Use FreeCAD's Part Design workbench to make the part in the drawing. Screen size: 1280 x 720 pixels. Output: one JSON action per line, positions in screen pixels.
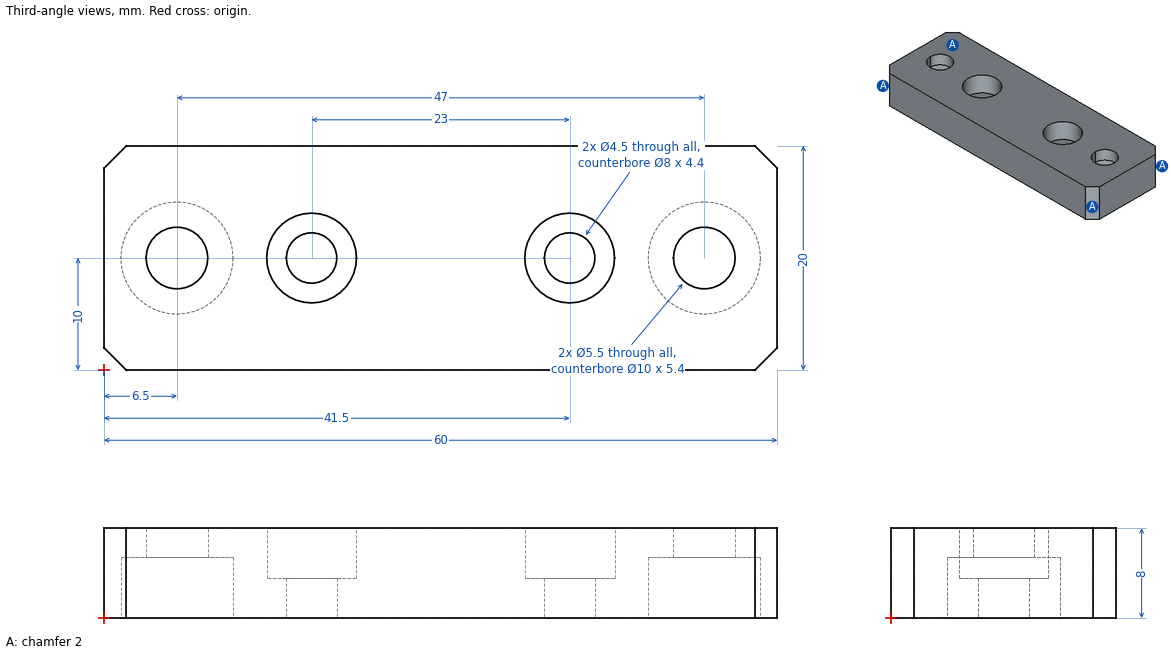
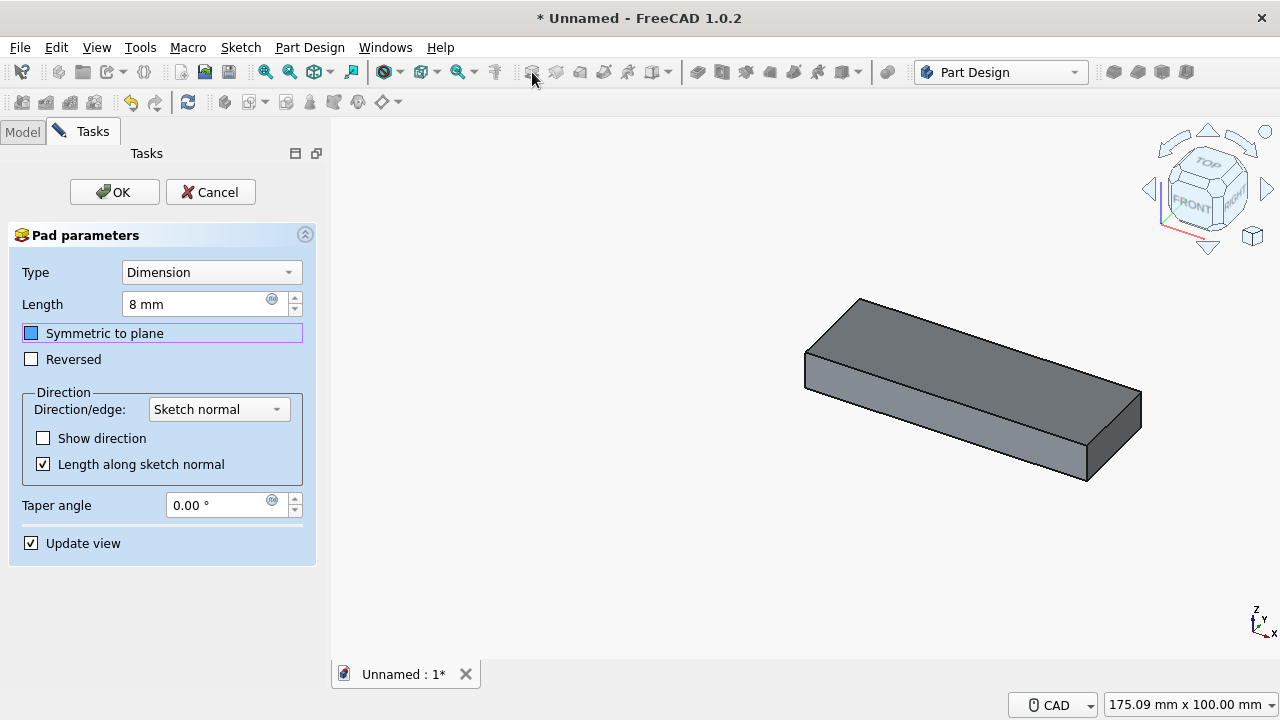
{"action": "left_click", "coordinate": [115, 192]}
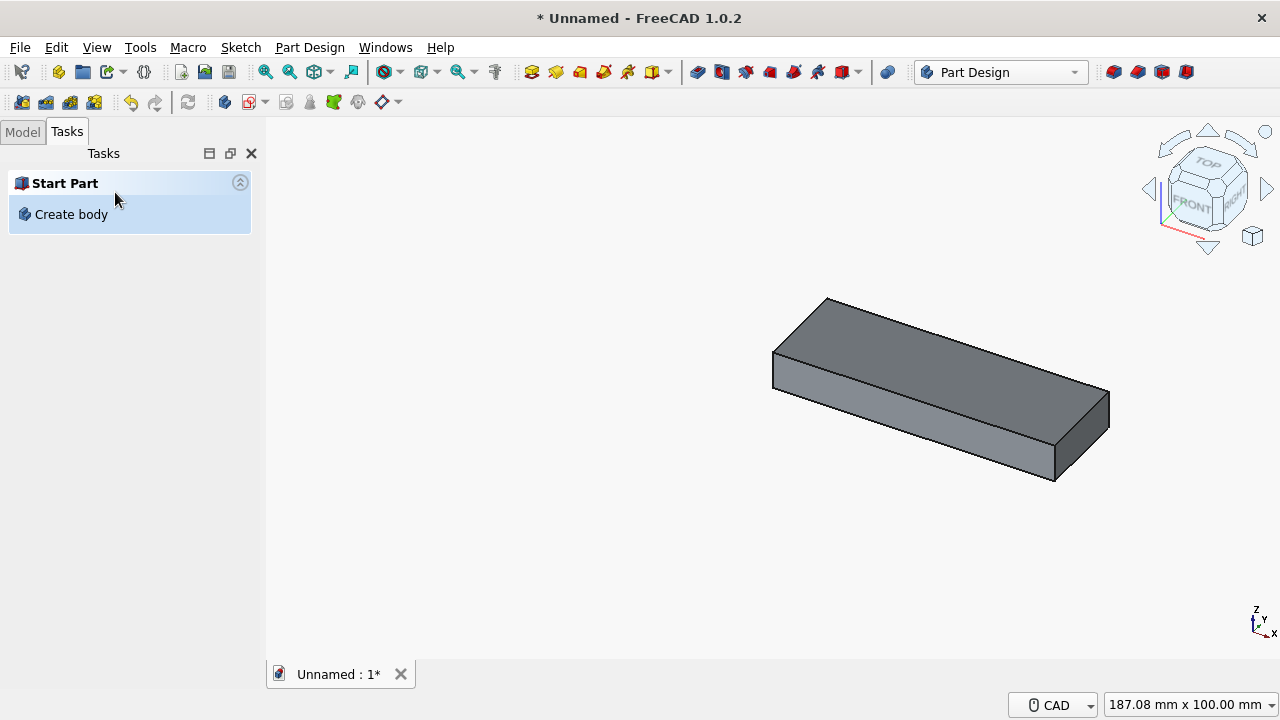
{"action": "key", "text": "v f"}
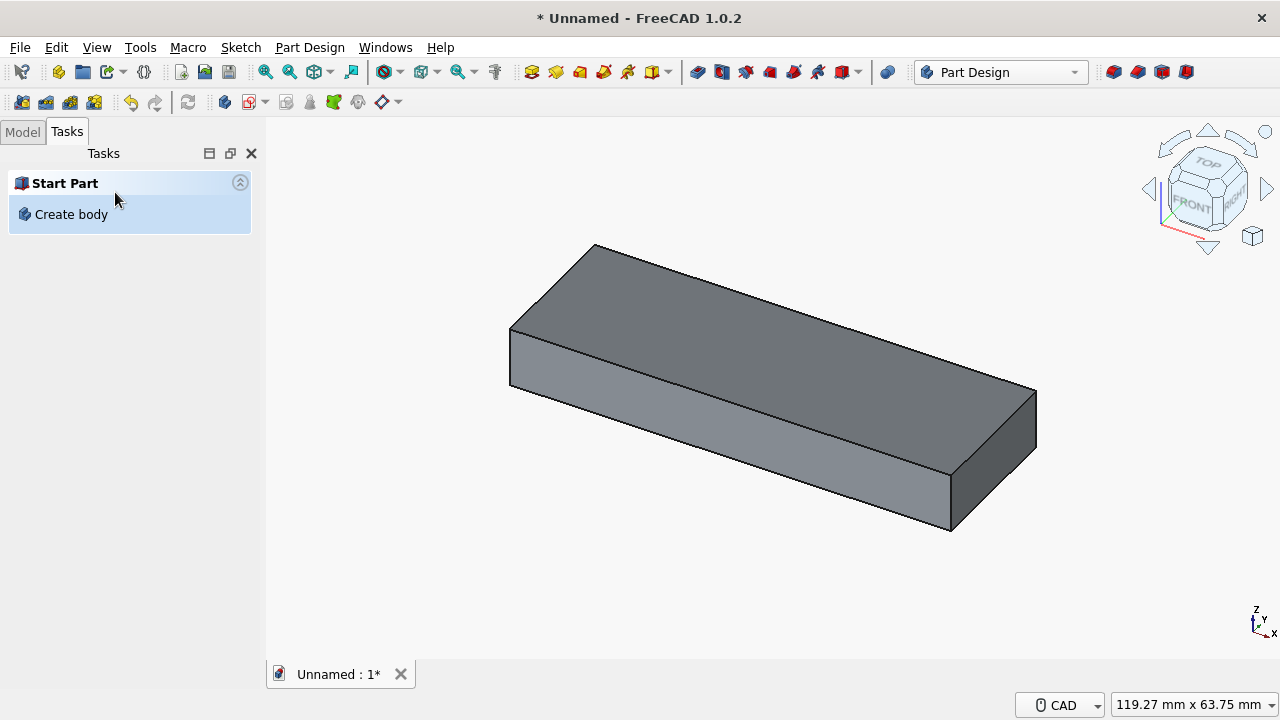
{"action": "left_click", "coordinate": [899, 401]}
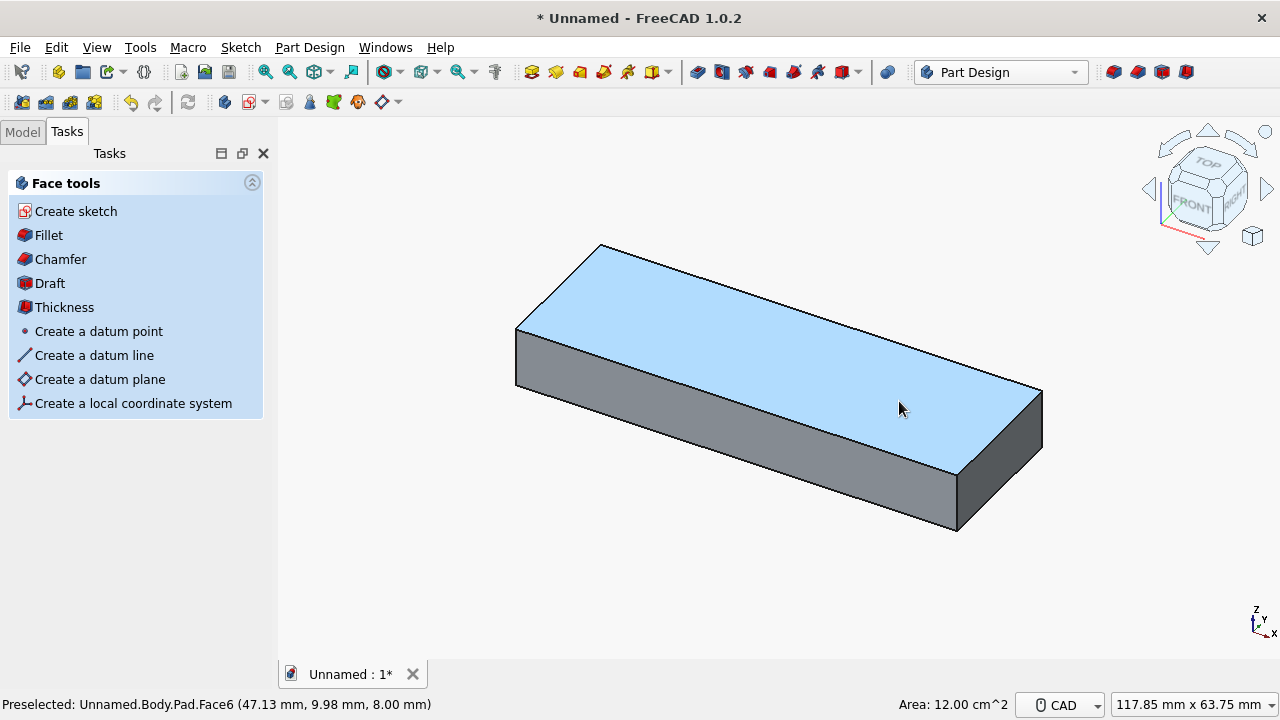
{"action": "left_click", "coordinate": [250, 102]}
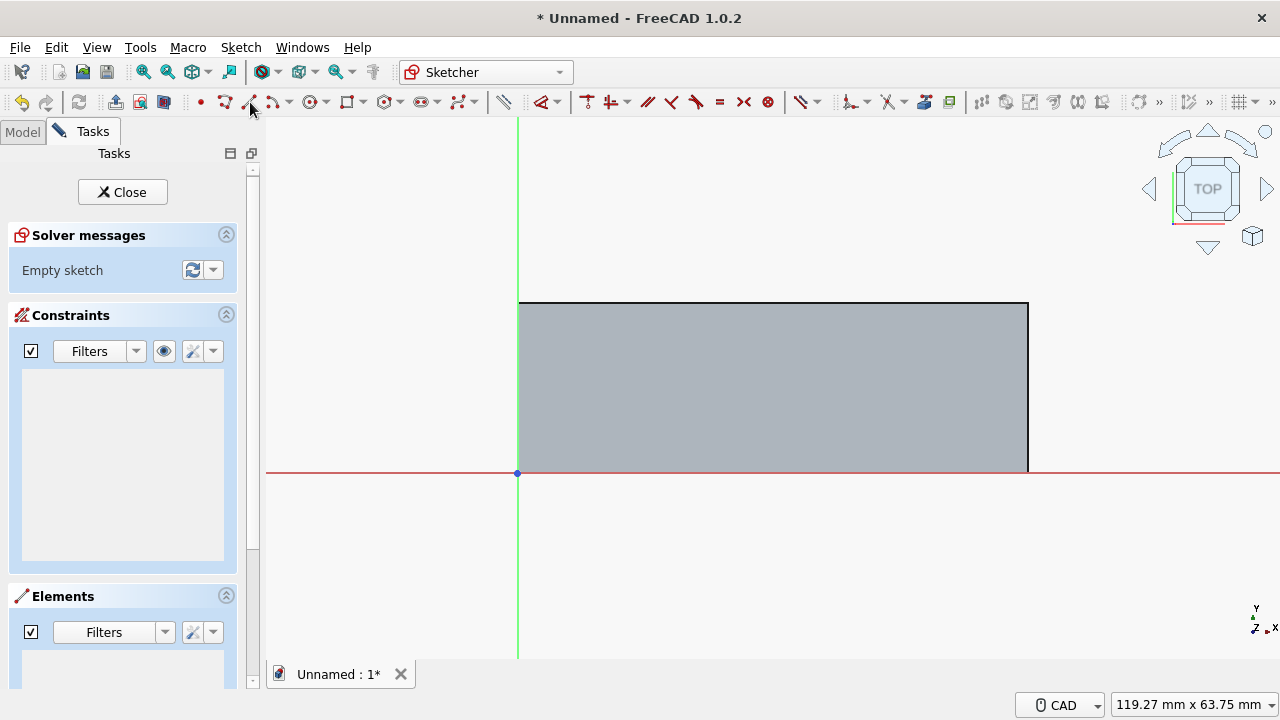
{"action": "scroll", "coordinate": [703, 488], "scroll_direction": "up", "scroll_amount": 2}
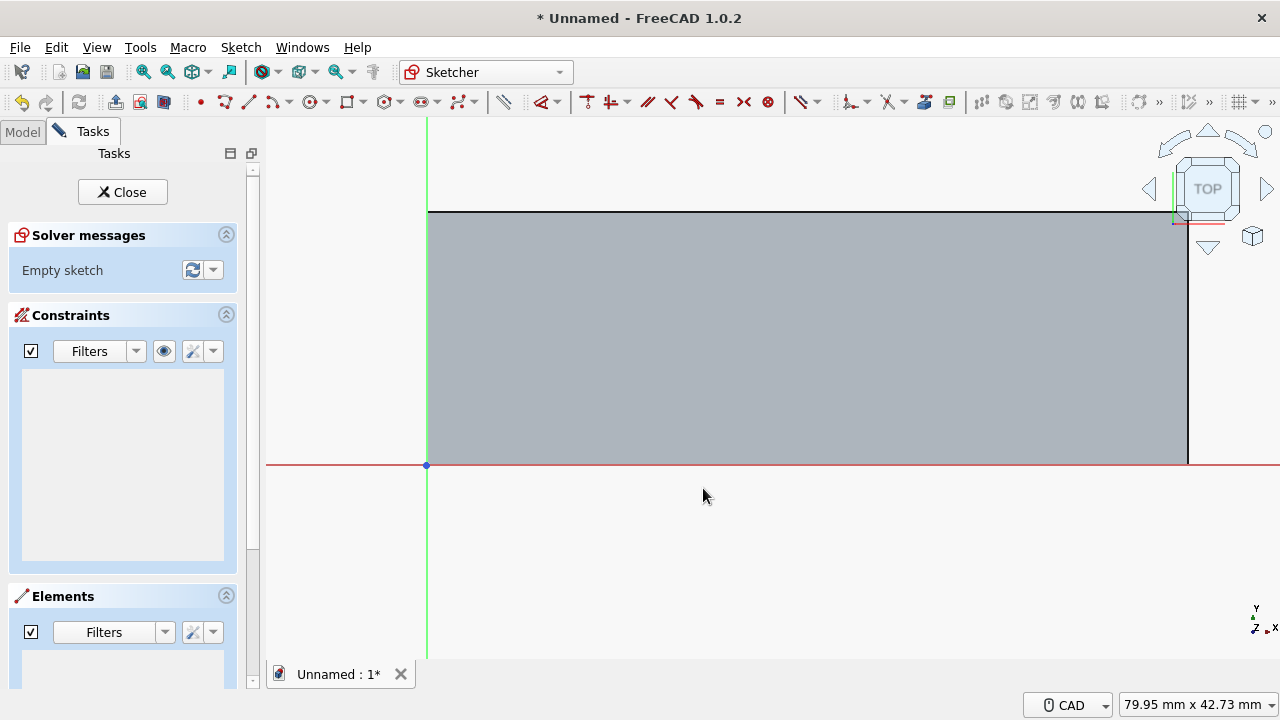
{"action": "left_click", "coordinate": [310, 102]}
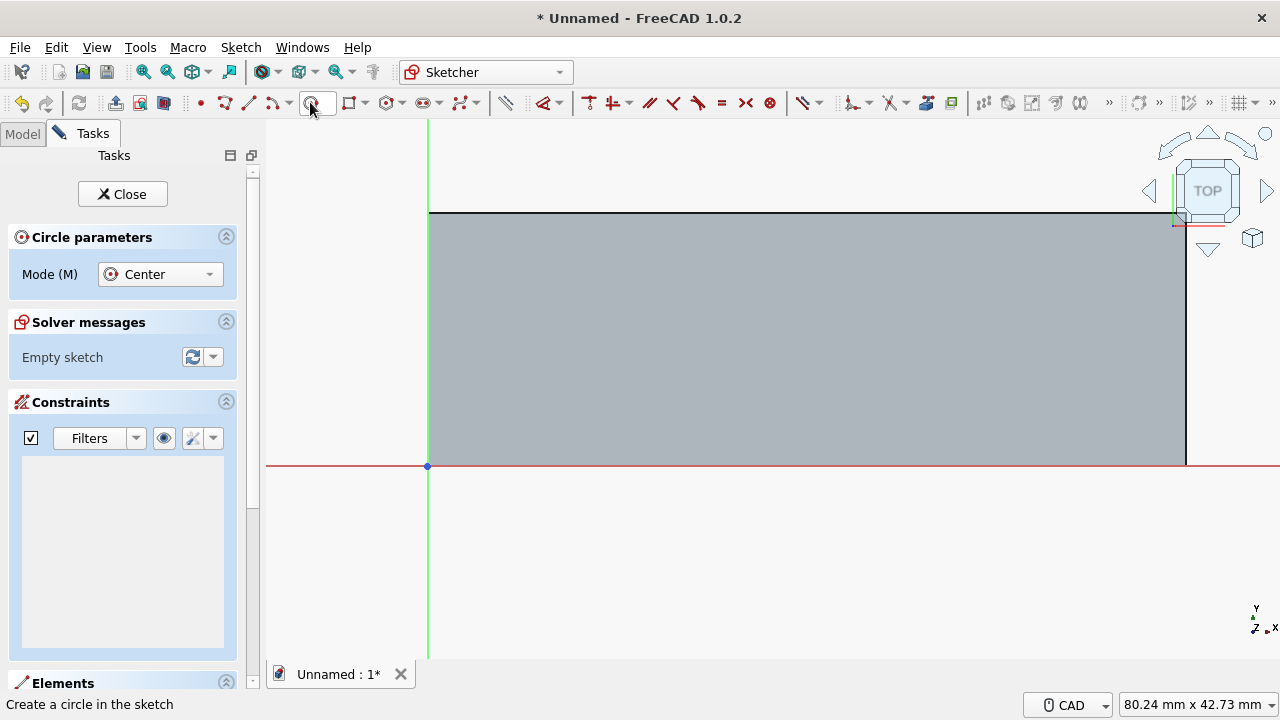
{"action": "left_click", "coordinate": [952, 340]}
{"action": "mouse_move", "coordinate": [973, 320]}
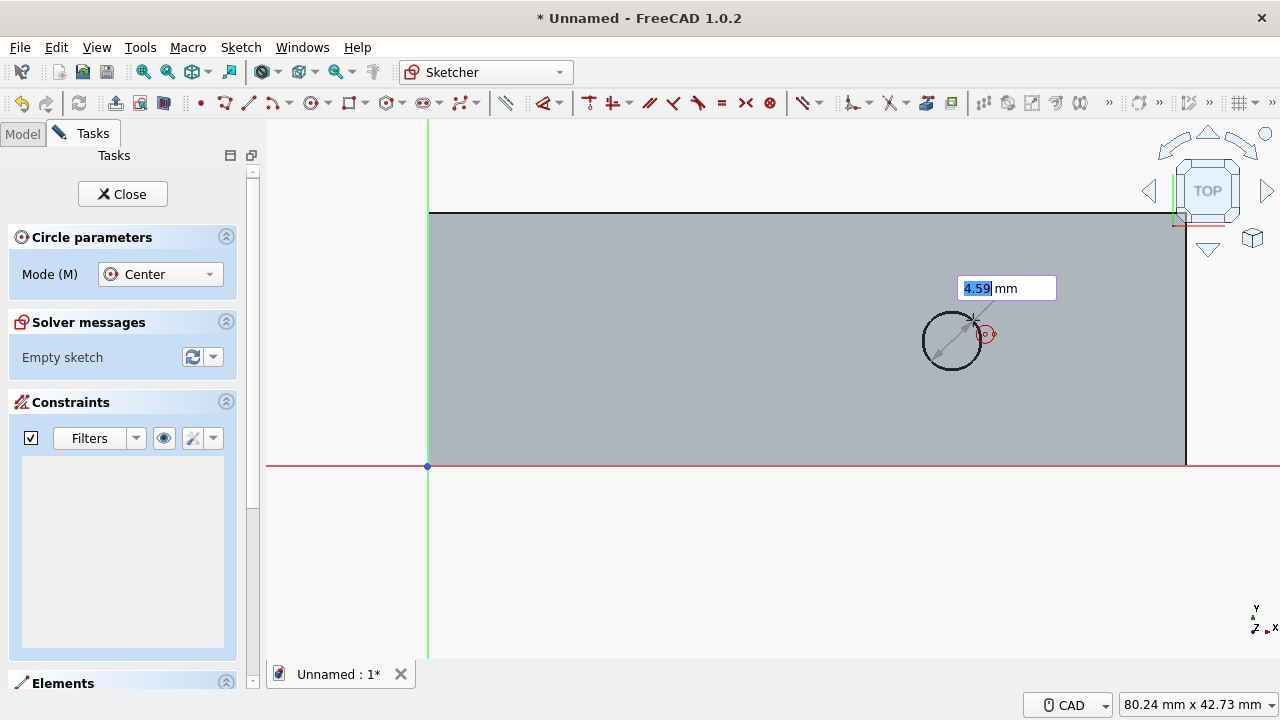
{"action": "type", "text": "4.5"}
{"action": "key", "text": "Return"}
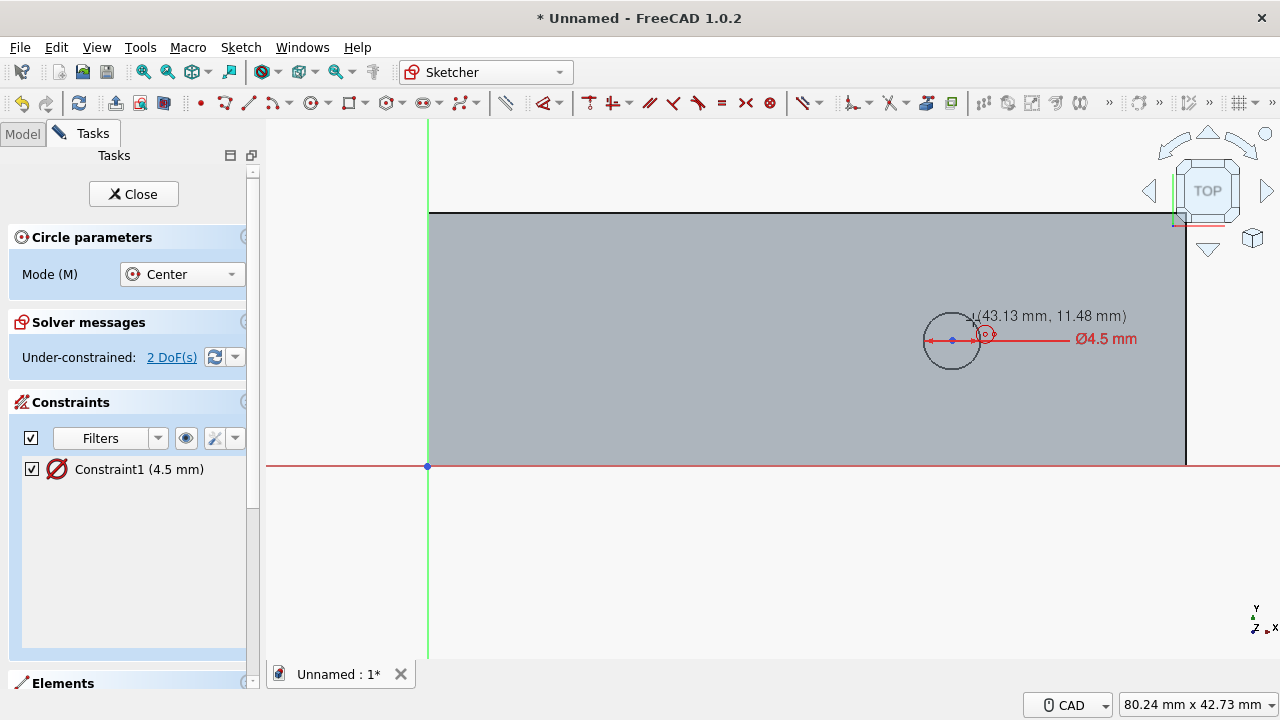
{"action": "left_click", "coordinate": [662, 340]}
{"action": "mouse_move", "coordinate": [682, 320]}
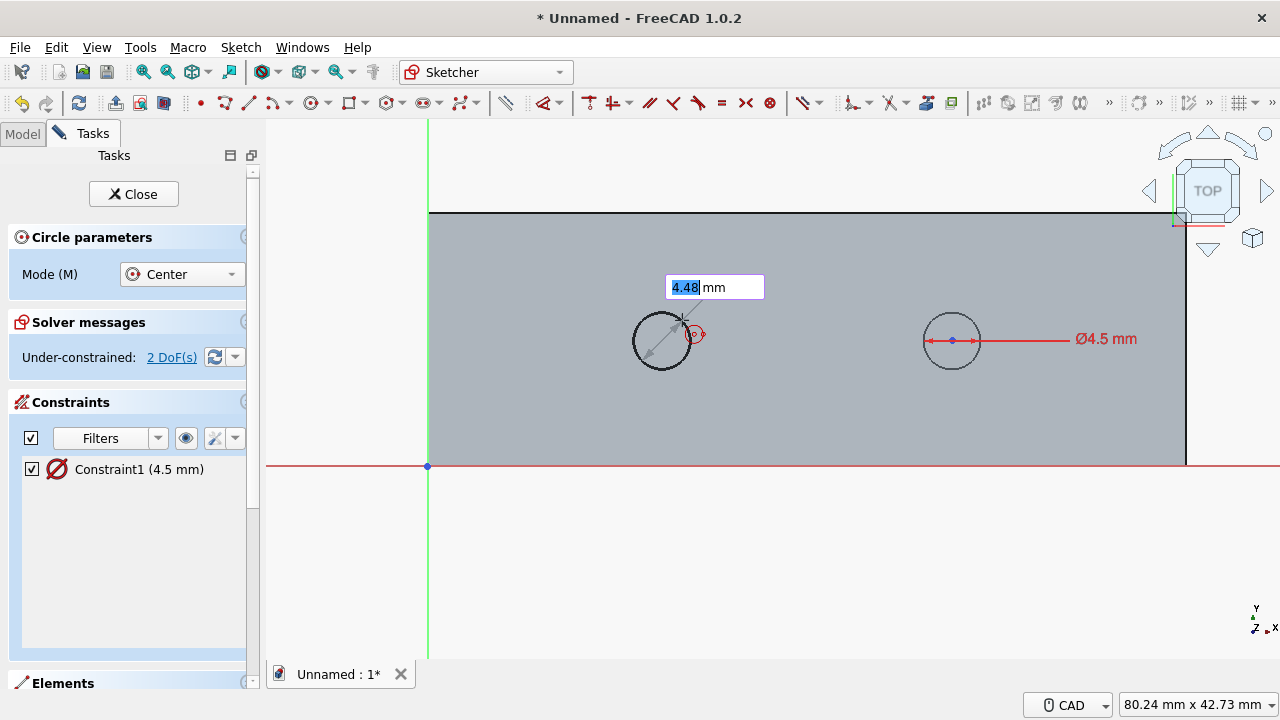
{"action": "type", "text": "4.5"}
{"action": "key", "text": "Return"}
{"action": "key", "text": "Escape"}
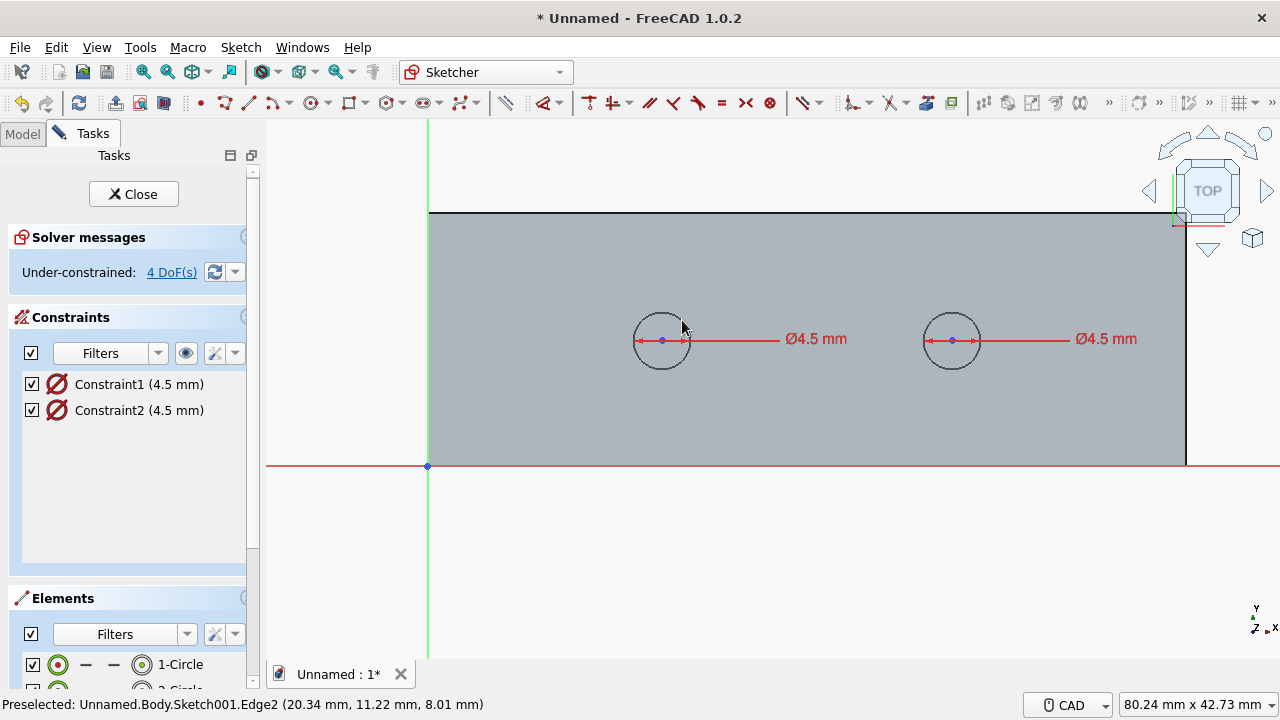
{"action": "left_click", "coordinate": [952, 341]}